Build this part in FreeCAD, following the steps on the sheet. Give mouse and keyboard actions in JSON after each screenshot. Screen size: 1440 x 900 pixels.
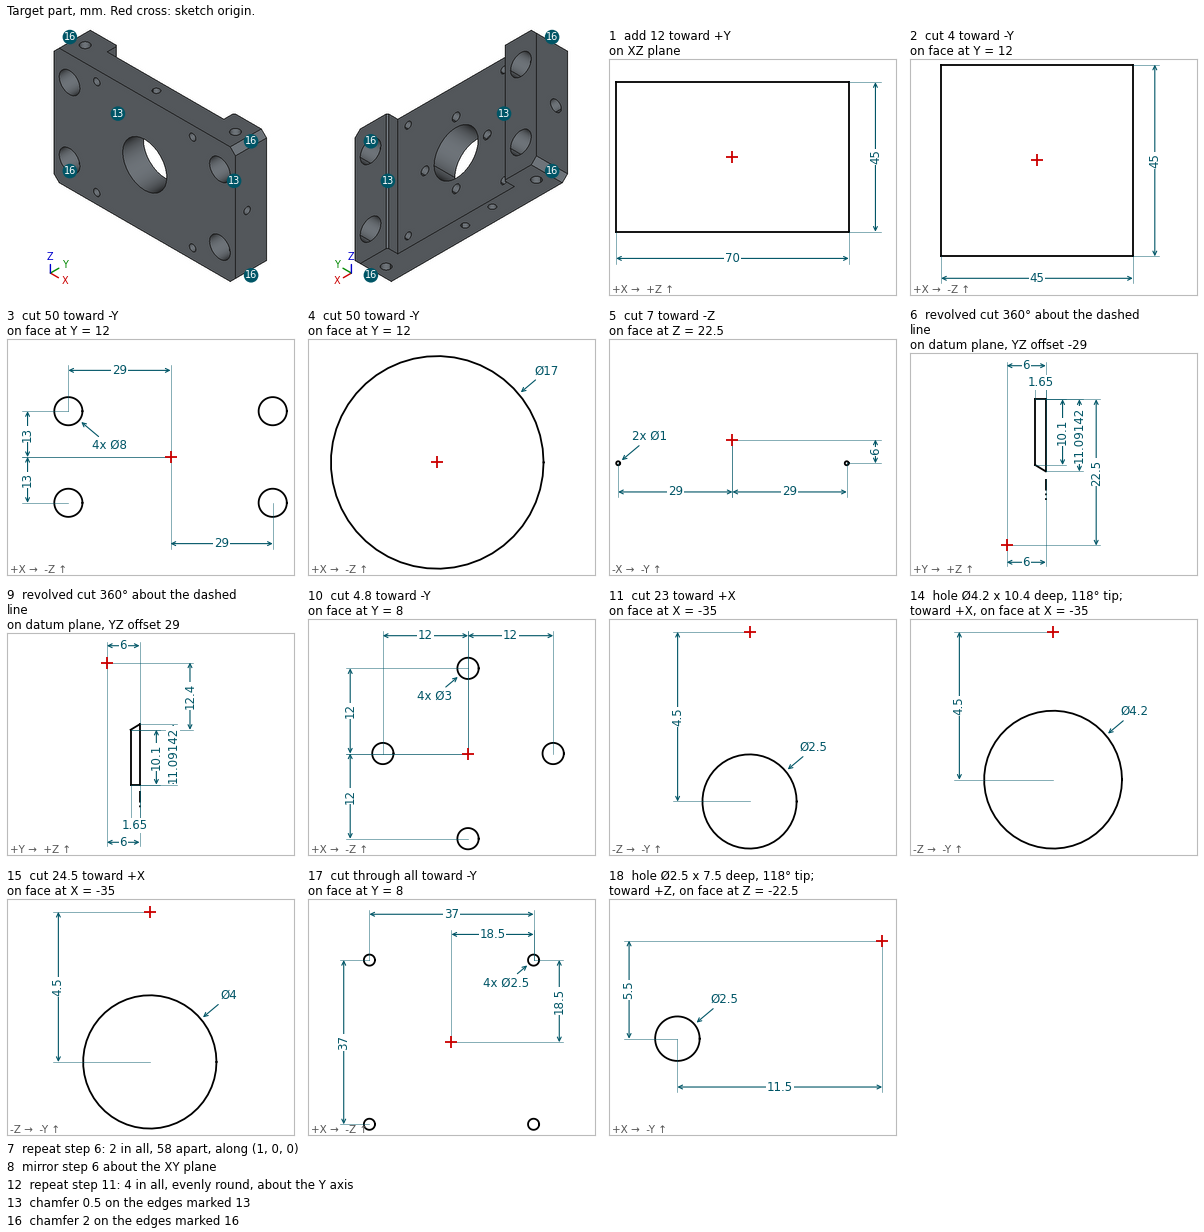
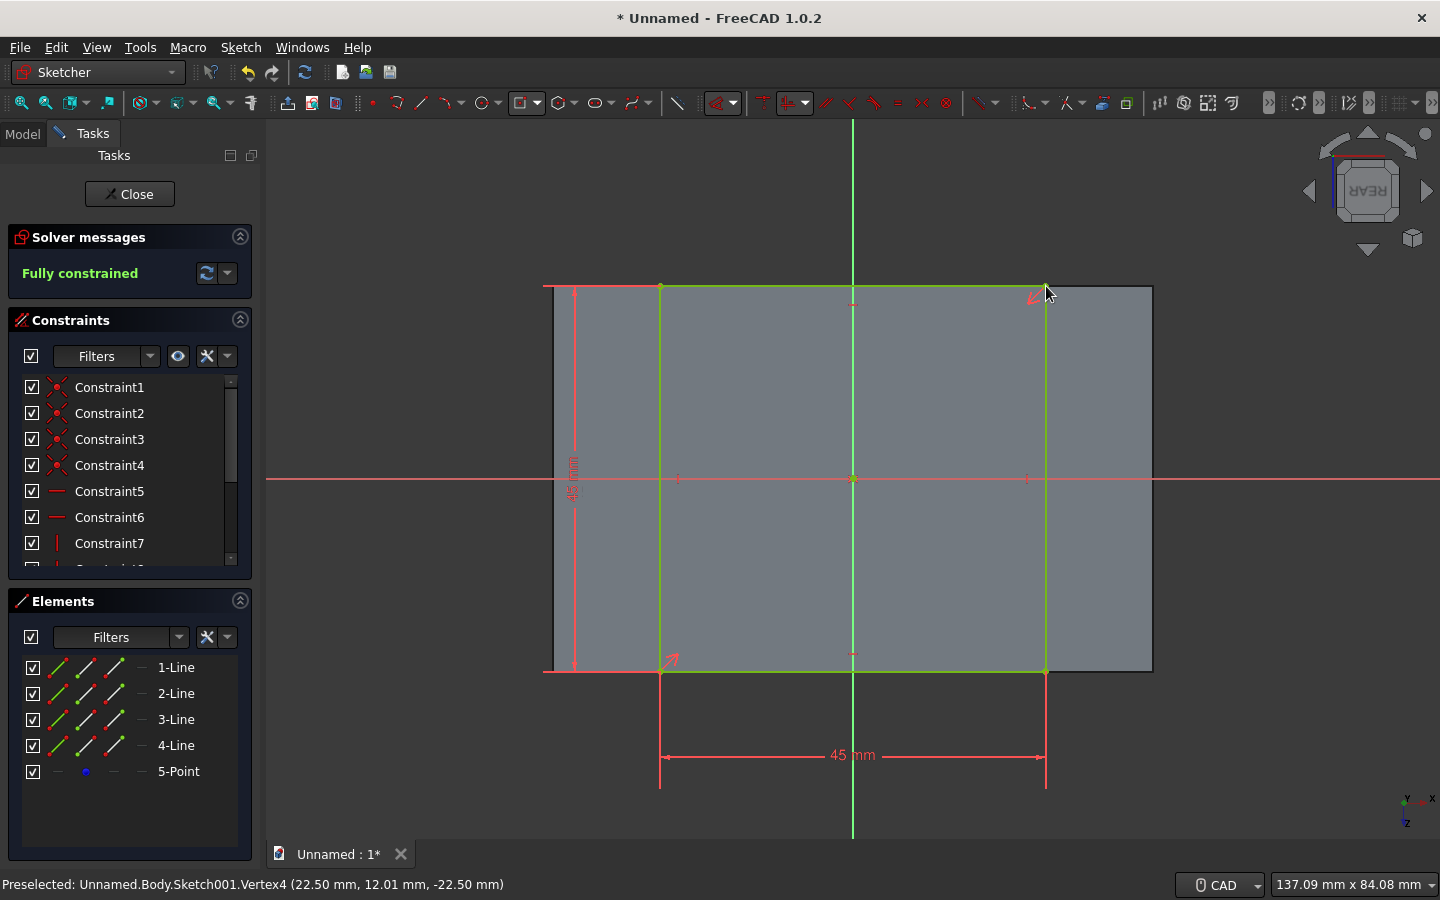
{"action": "left_click", "coordinate": [130, 194]}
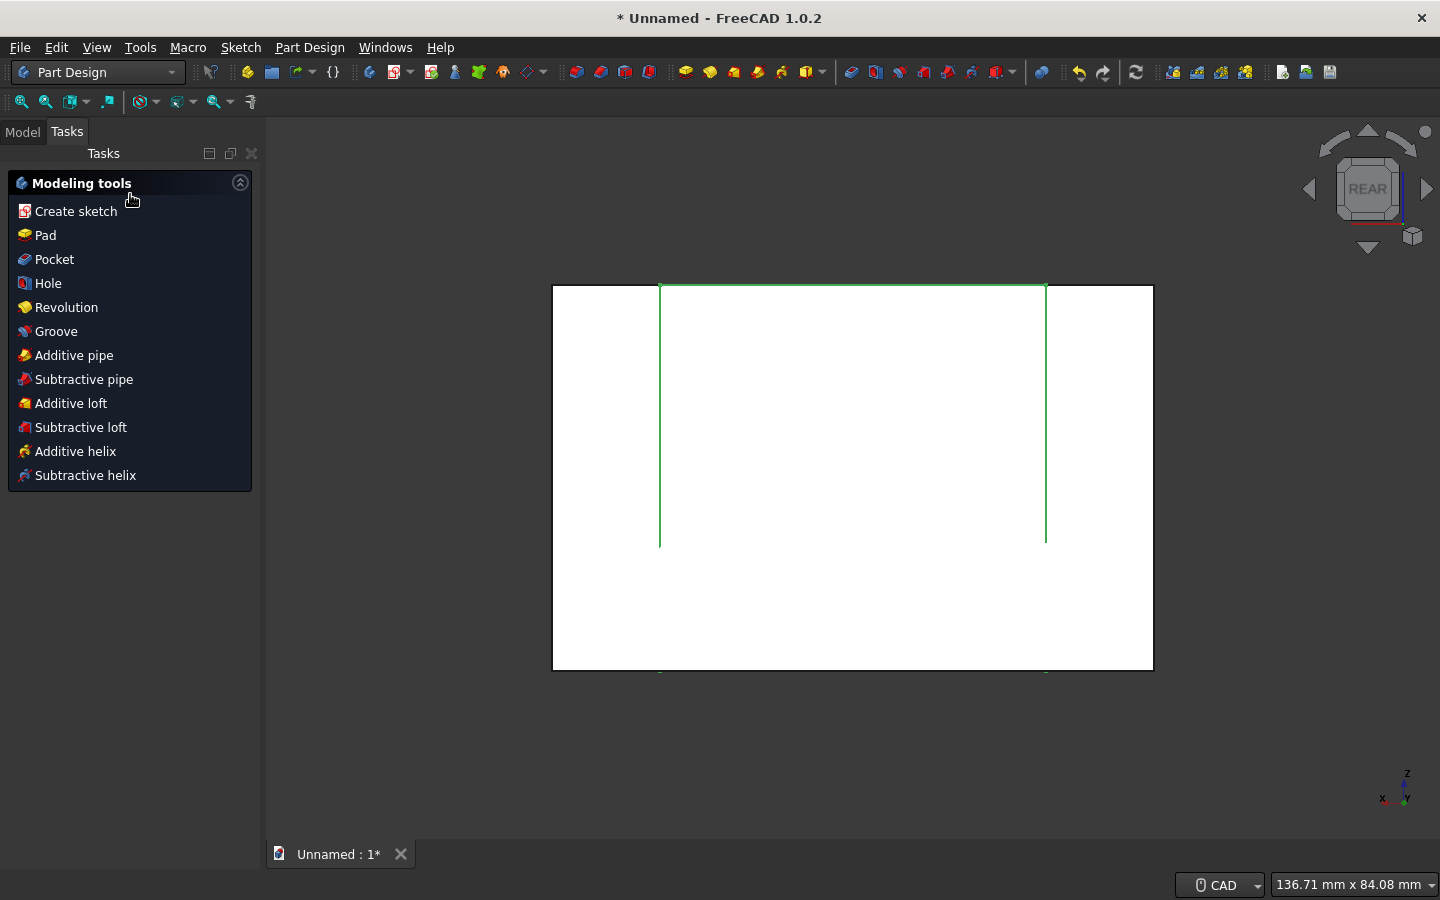
{"action": "left_click", "coordinate": [852, 72]}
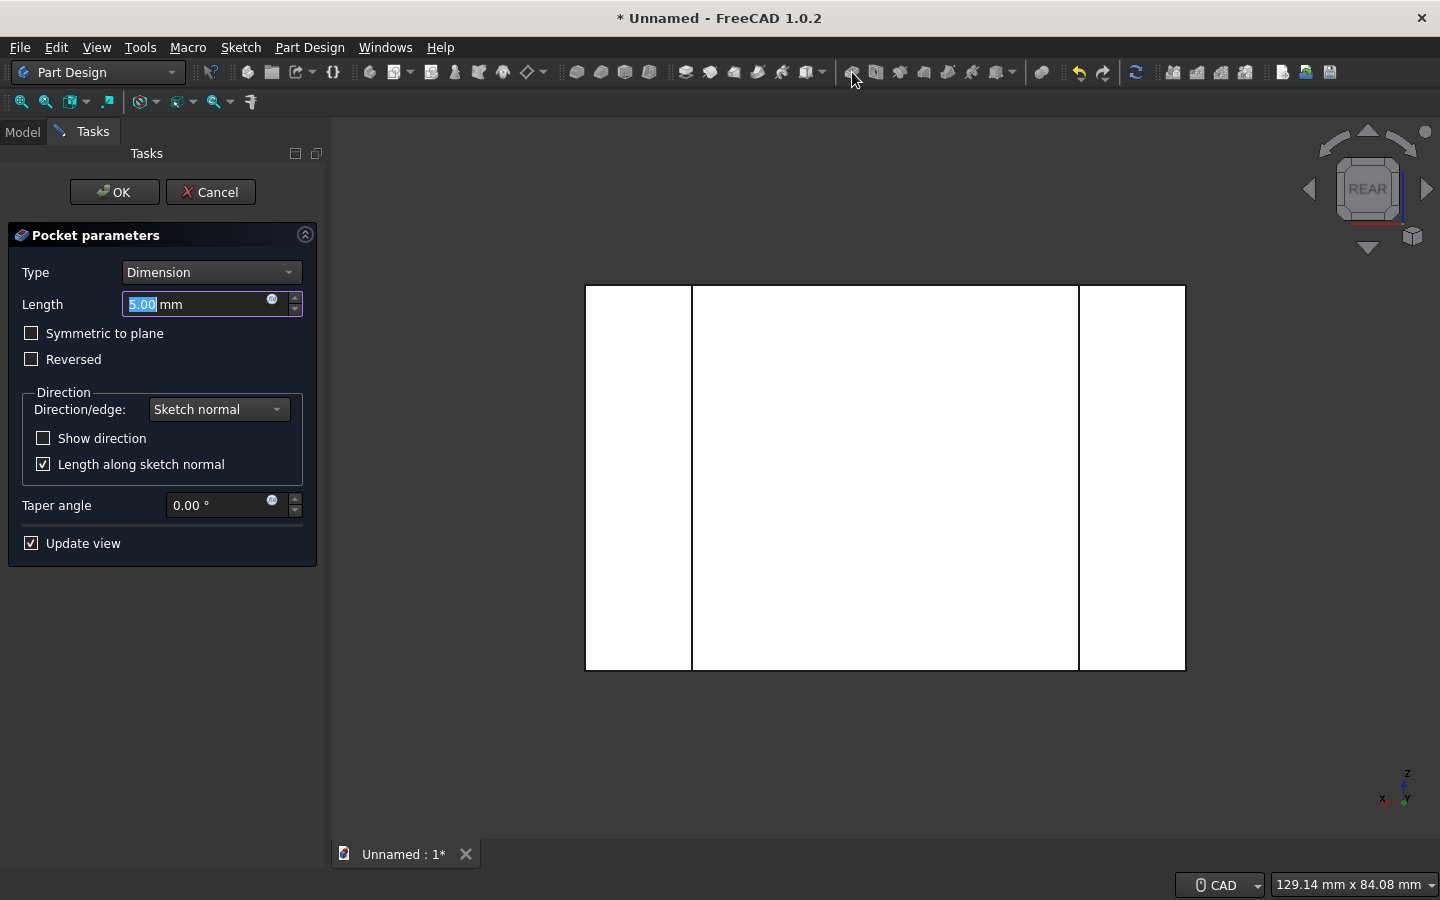
{"action": "type", "text": "4"}
{"action": "key", "text": "Tab"}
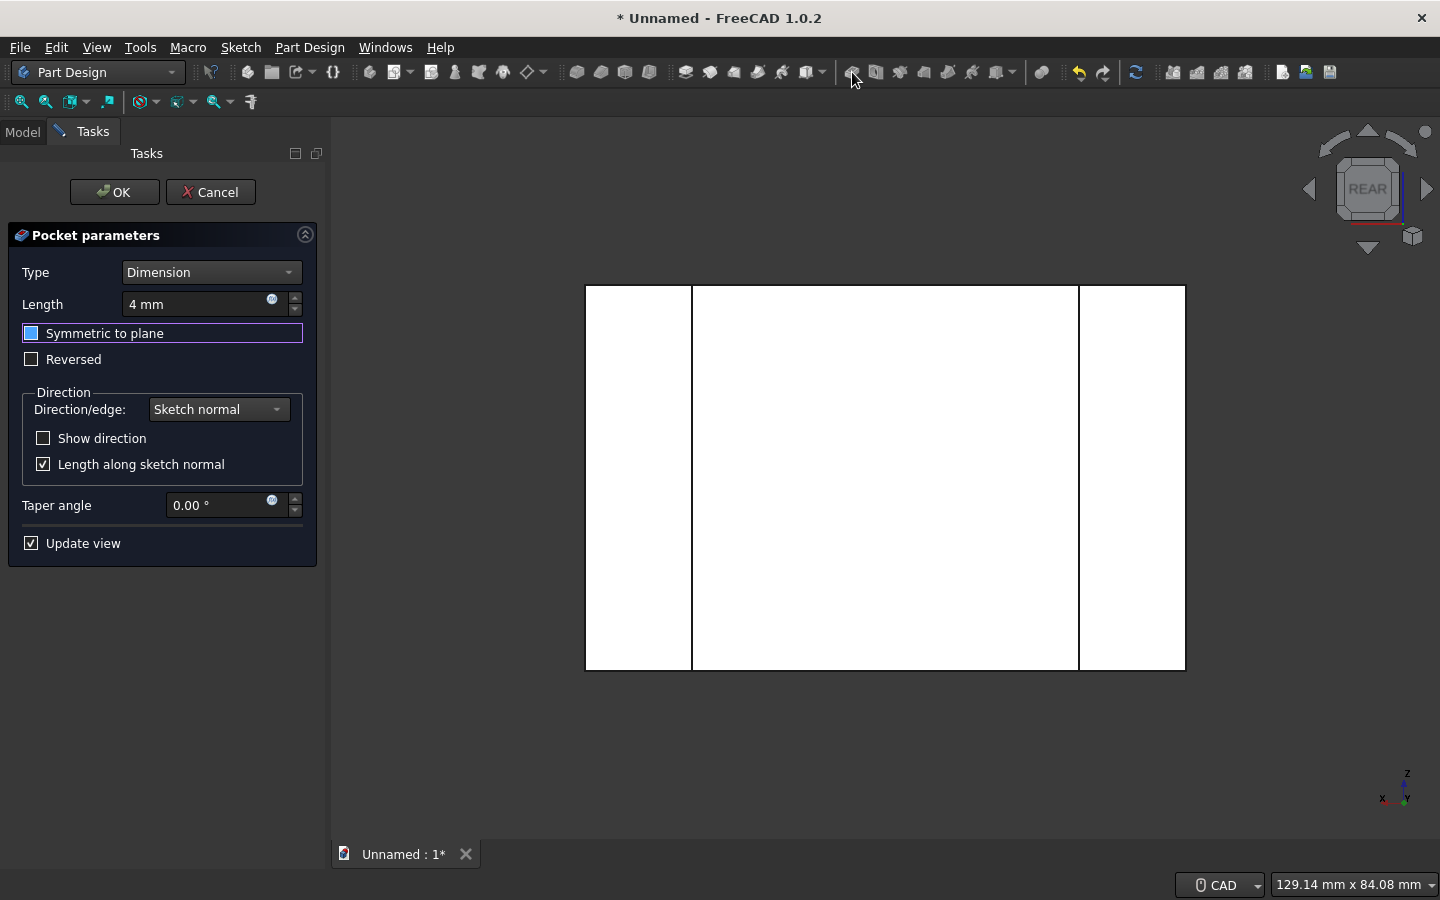
{"action": "left_click", "coordinate": [115, 192]}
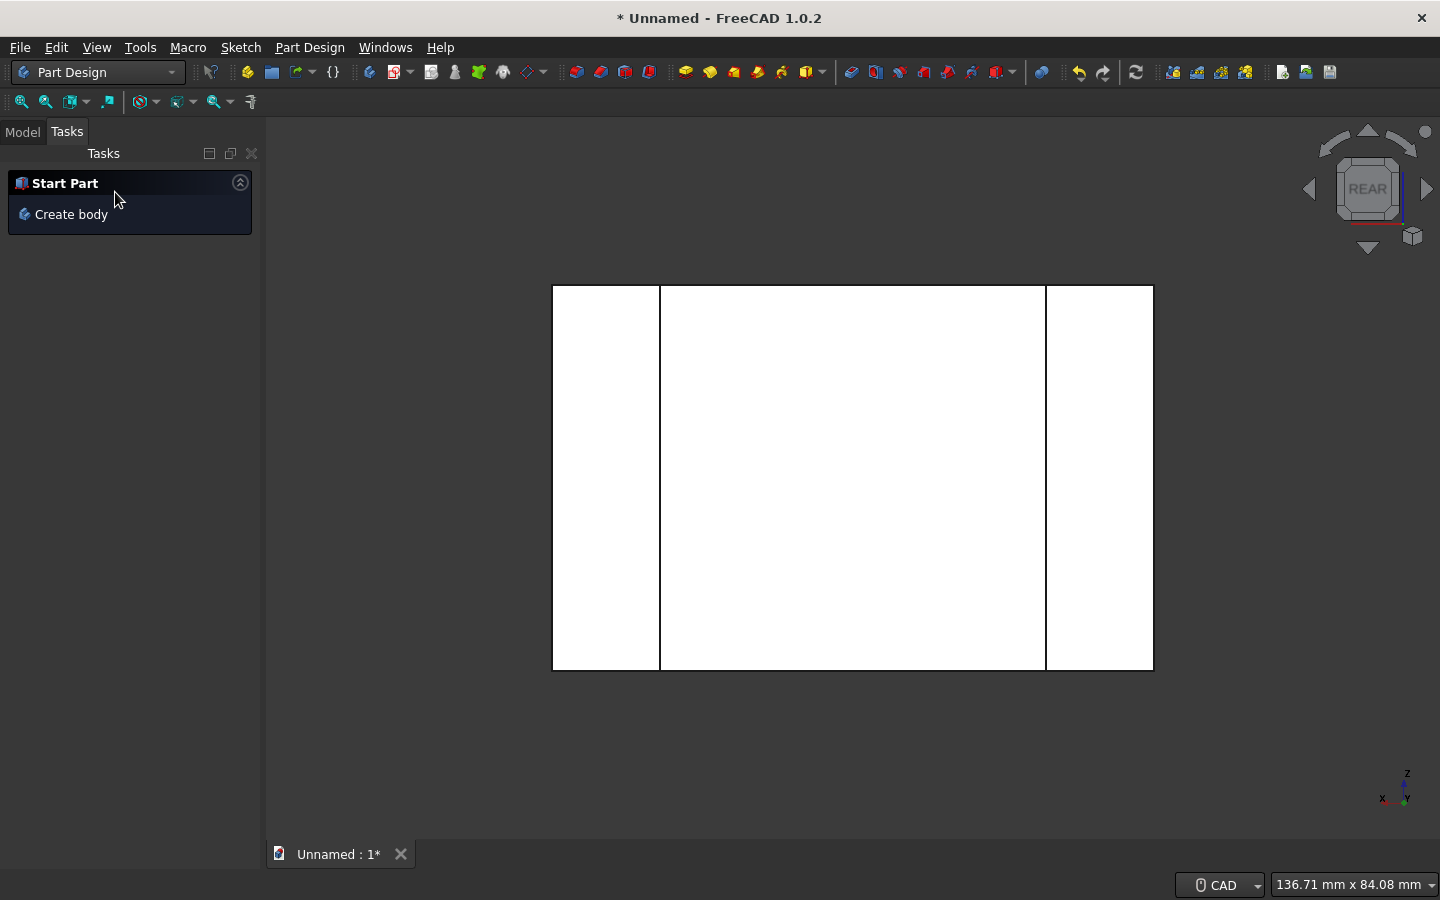
{"action": "left_click", "coordinate": [606, 367]}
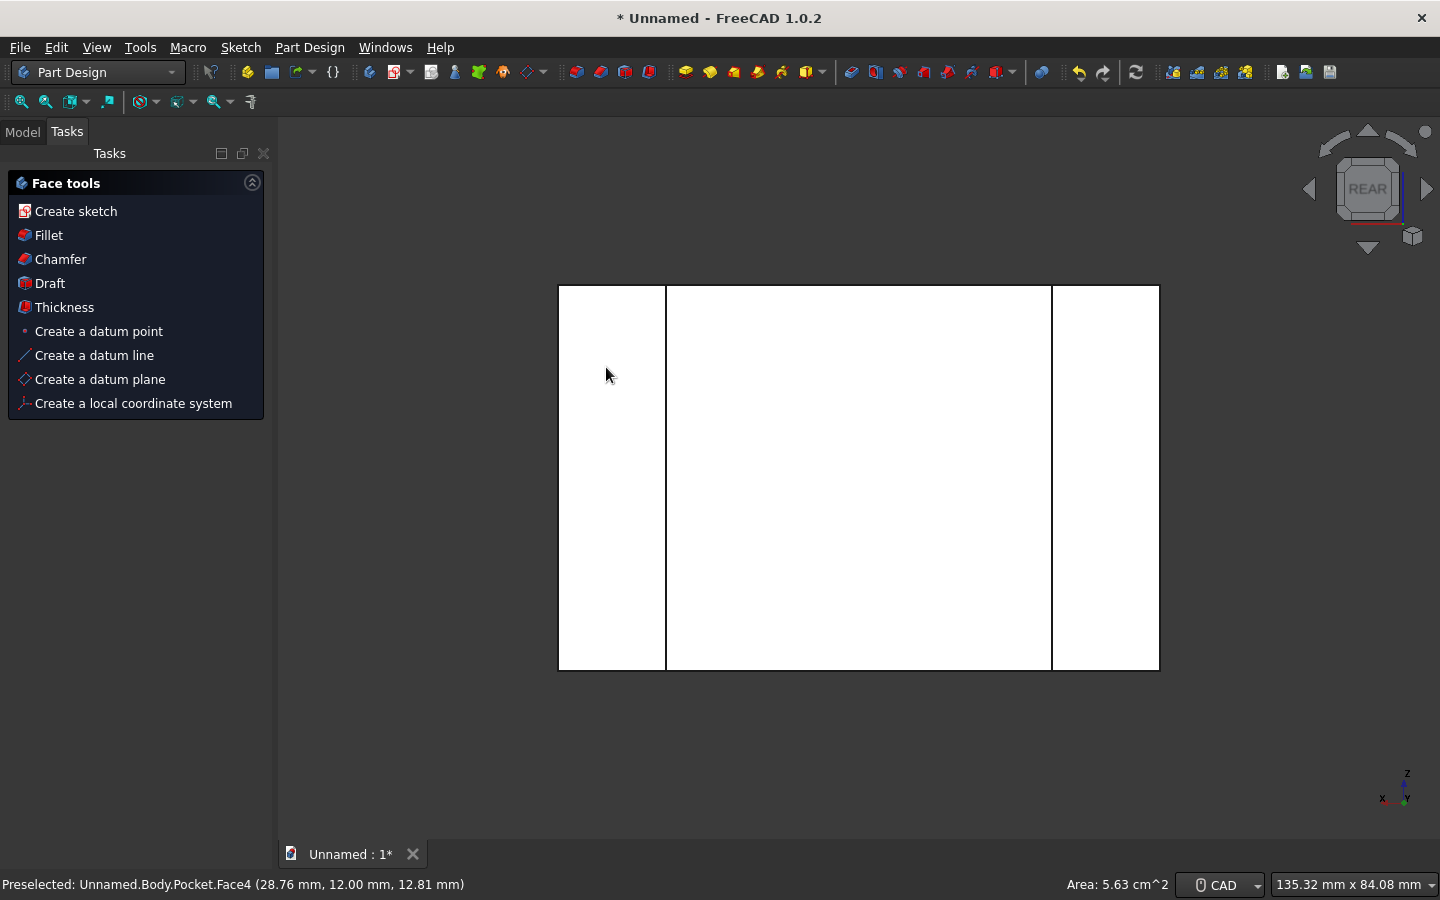
{"action": "left_click", "coordinate": [394, 72]}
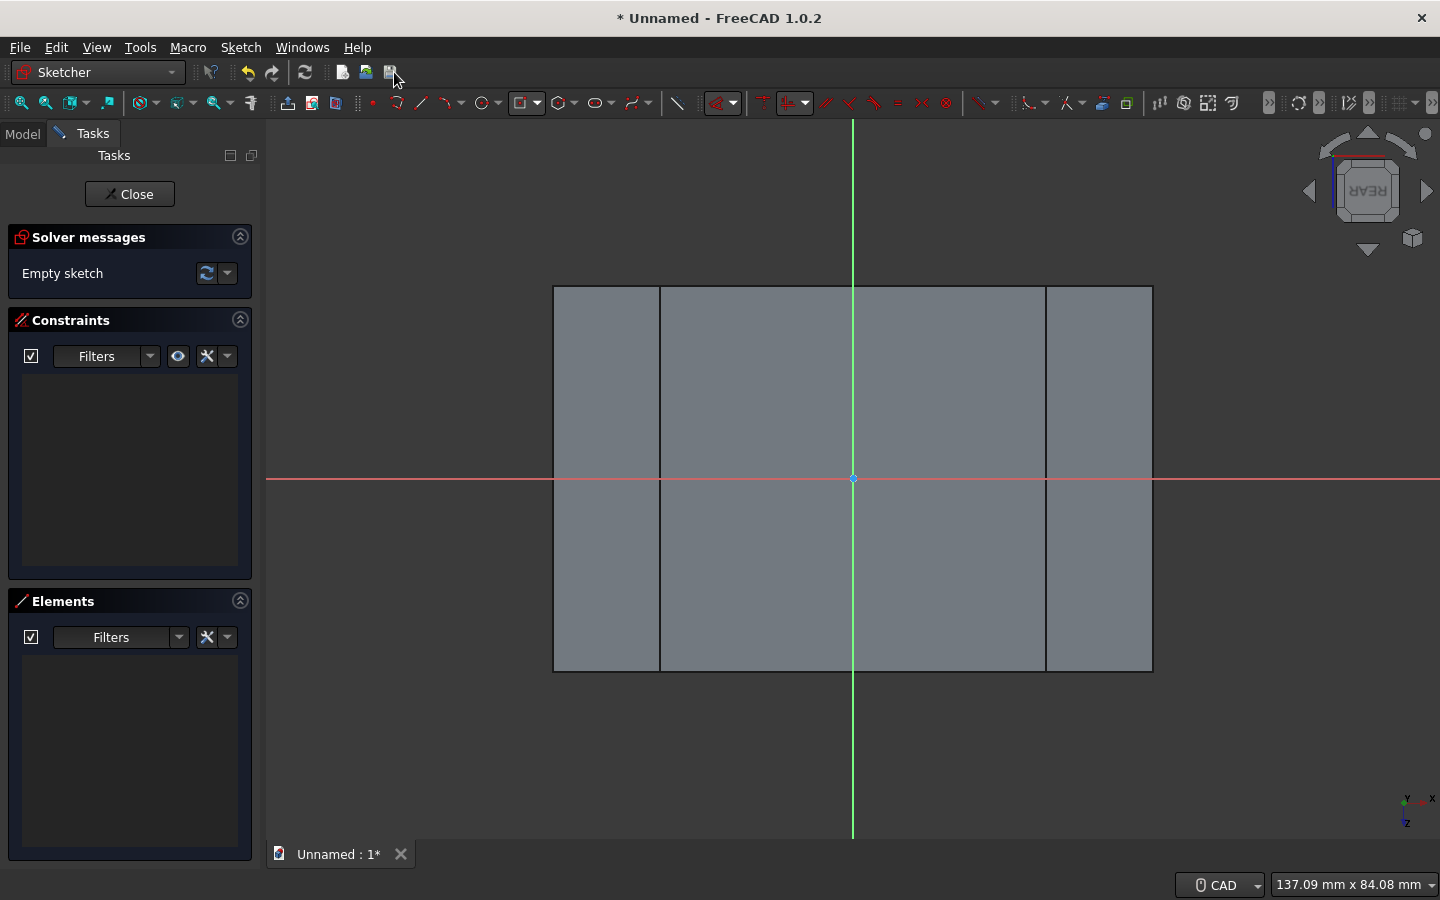
{"action": "left_click", "coordinate": [482, 104]}